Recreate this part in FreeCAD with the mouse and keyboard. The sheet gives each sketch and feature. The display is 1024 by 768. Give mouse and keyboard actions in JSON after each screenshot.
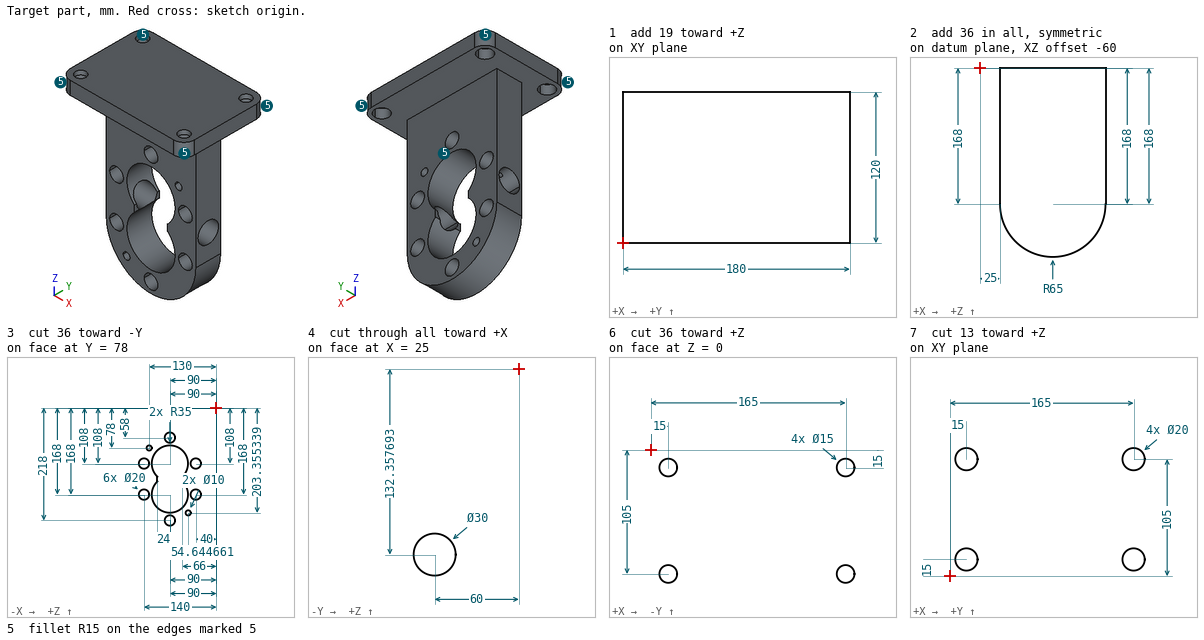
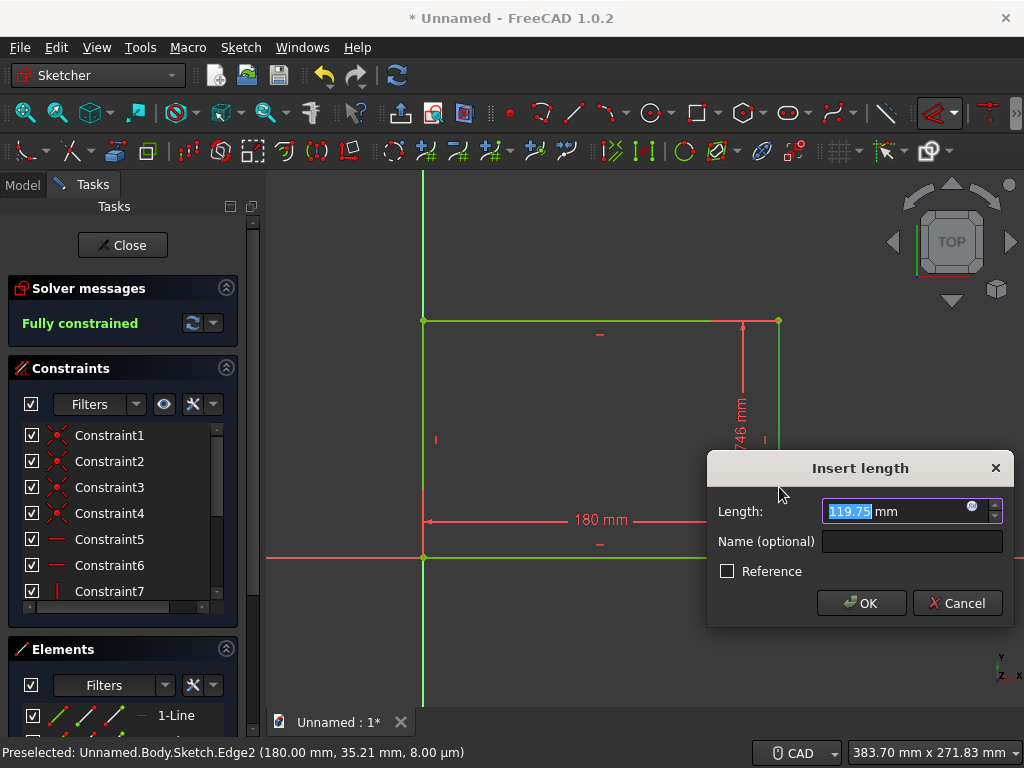
{"action": "type", "text": "120"}
{"action": "key", "text": "Return"}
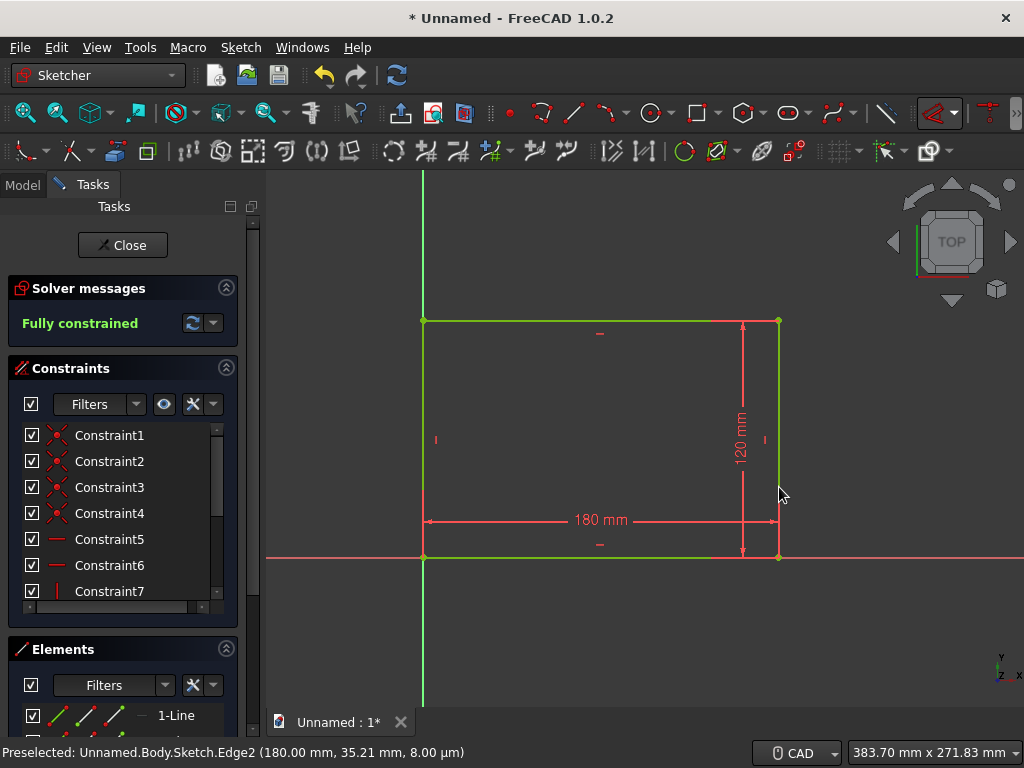
{"action": "left_click", "coordinate": [123, 245]}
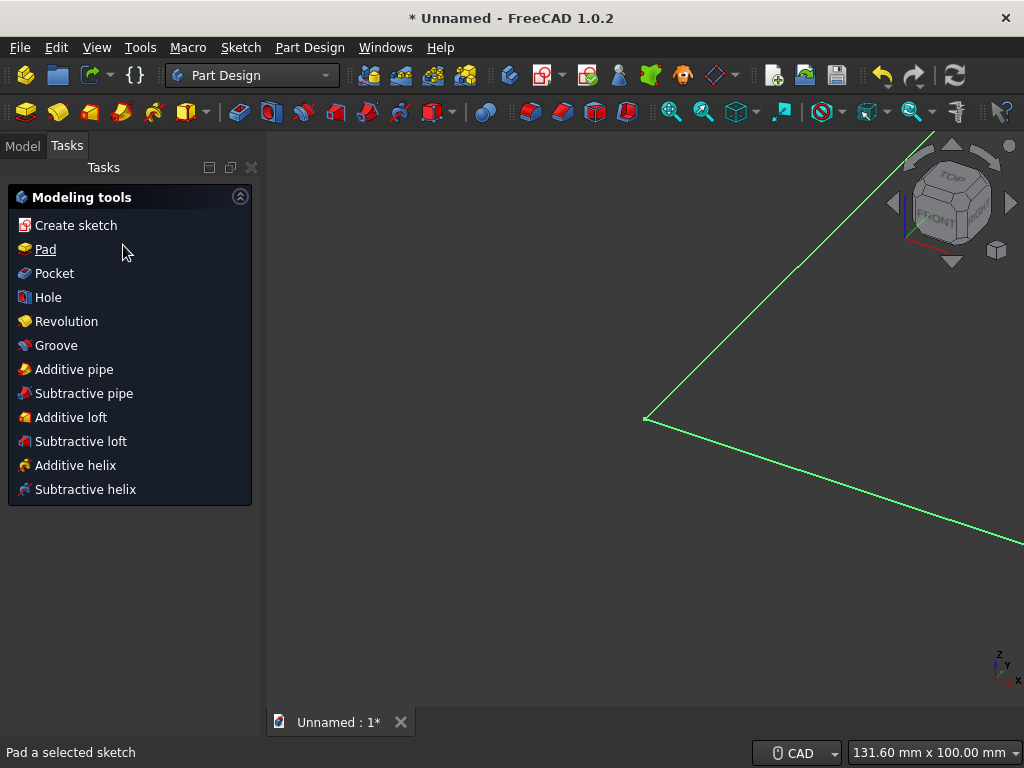
{"action": "left_click", "coordinate": [26, 112]}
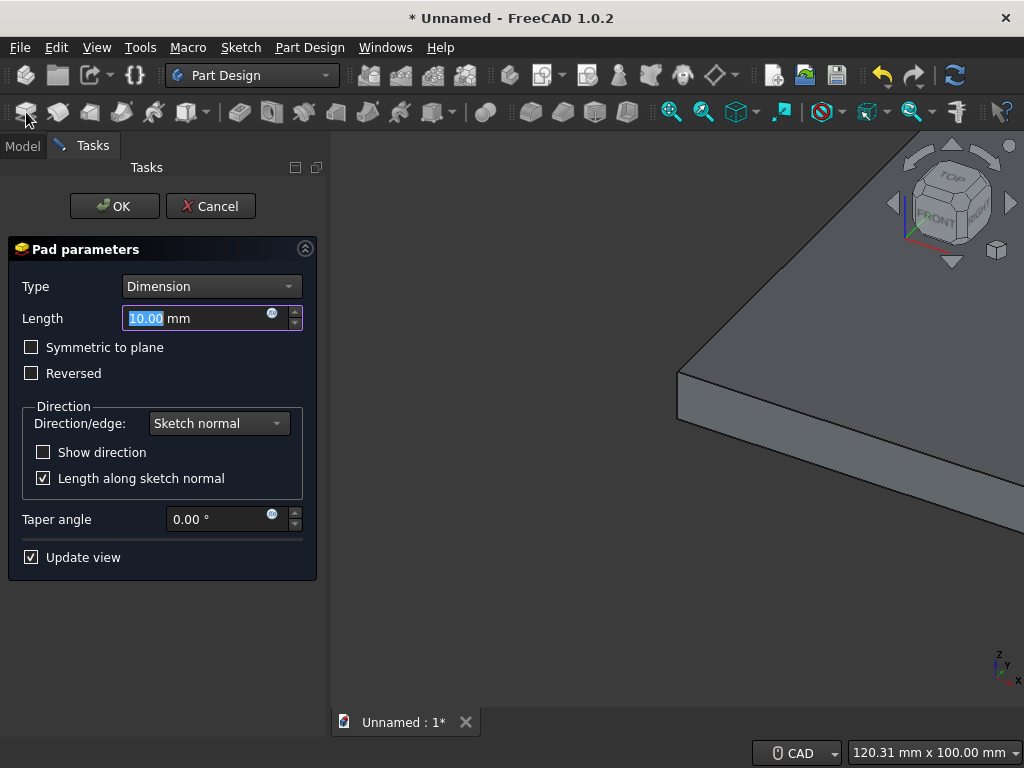
{"action": "type", "text": "19"}
{"action": "key", "text": "Tab"}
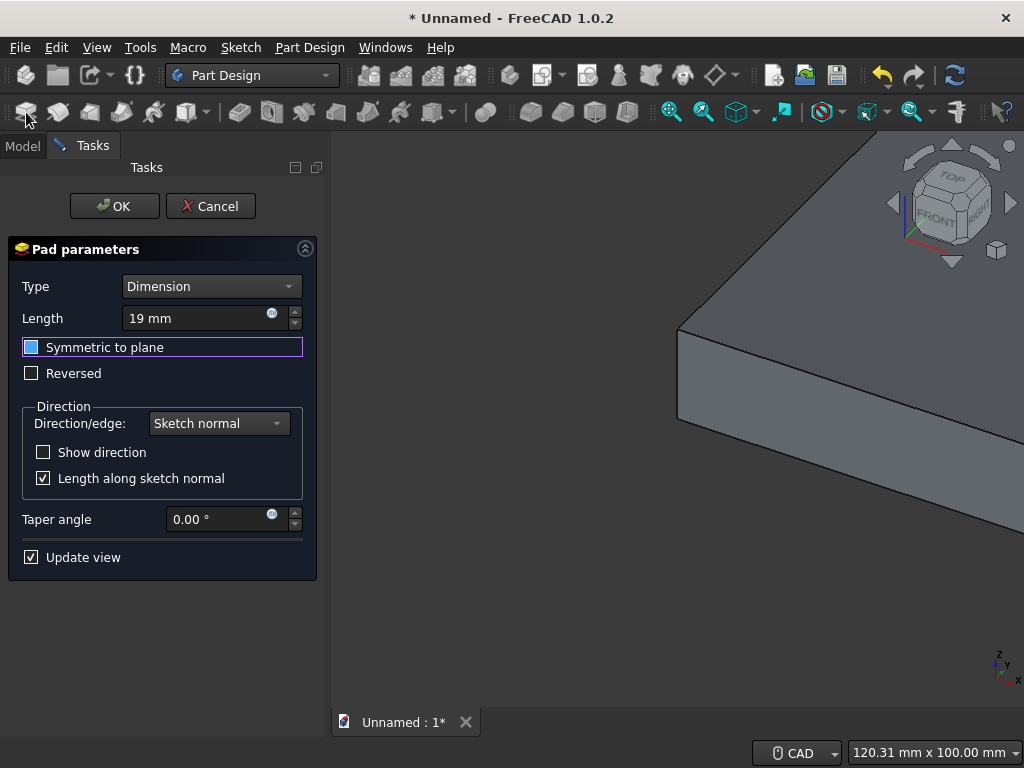
{"action": "left_click", "coordinate": [115, 206]}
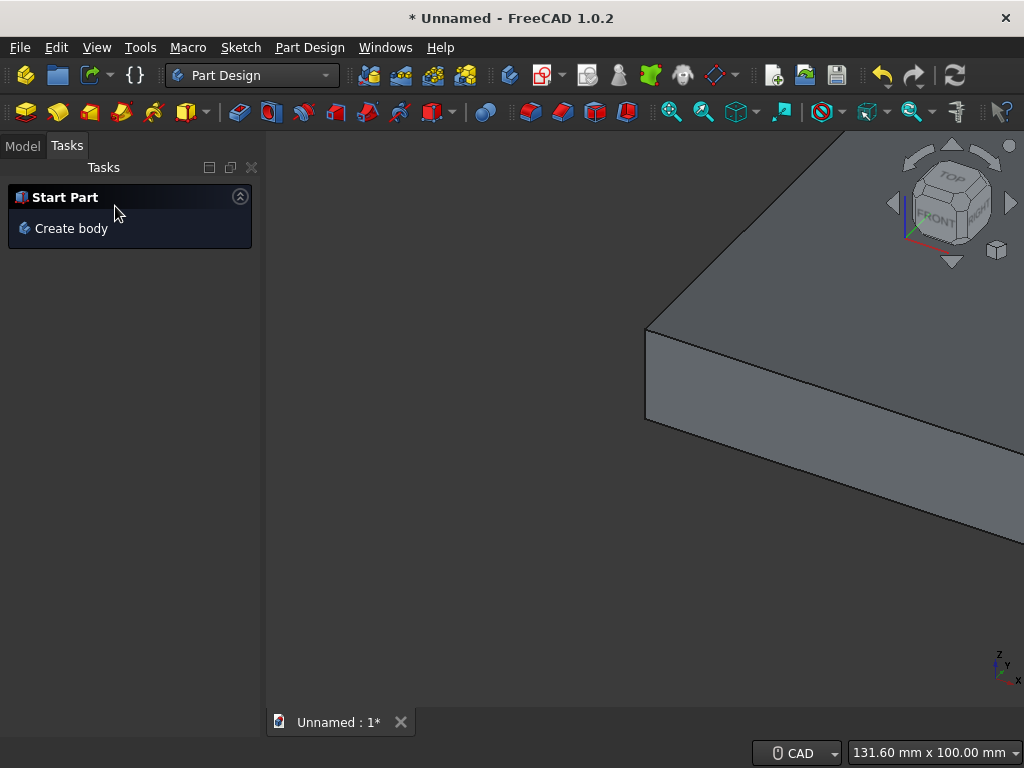
{"action": "left_click", "coordinate": [672, 112]}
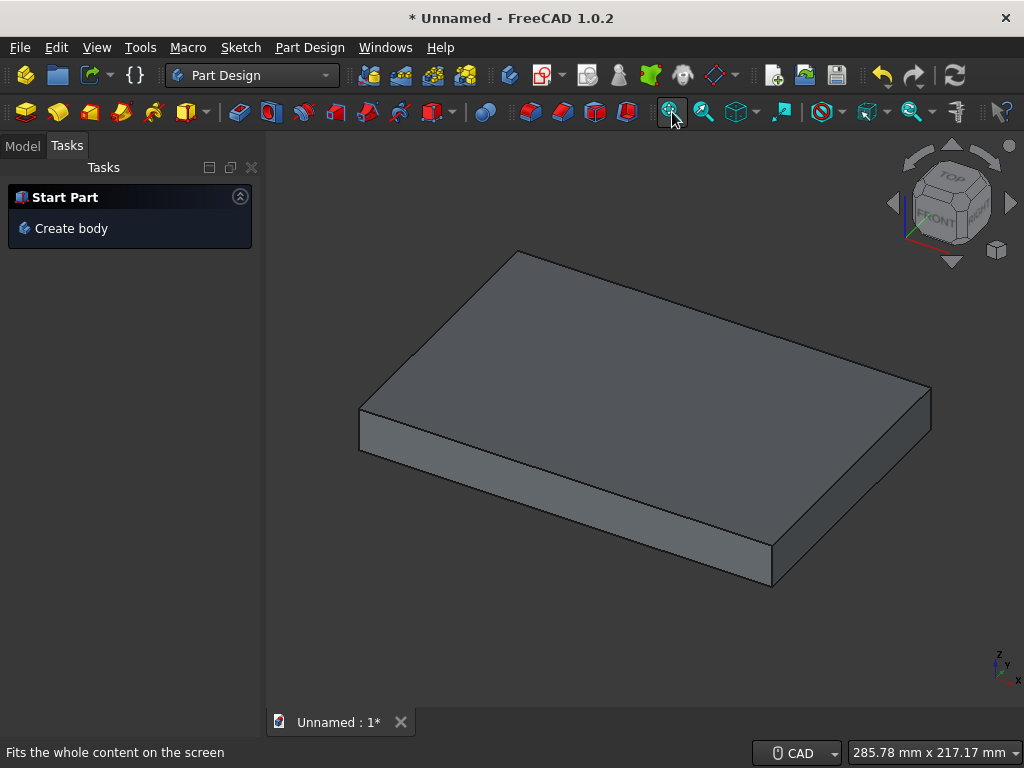
{"action": "left_click", "coordinate": [23, 145]}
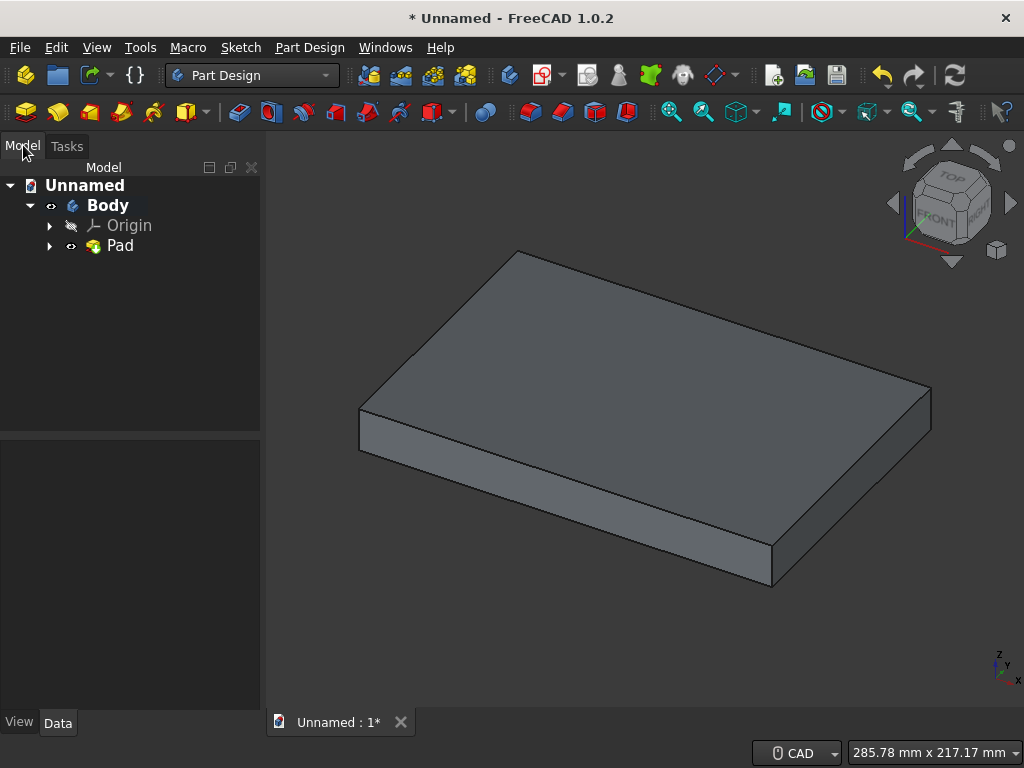
{"action": "left_click", "coordinate": [50, 226]}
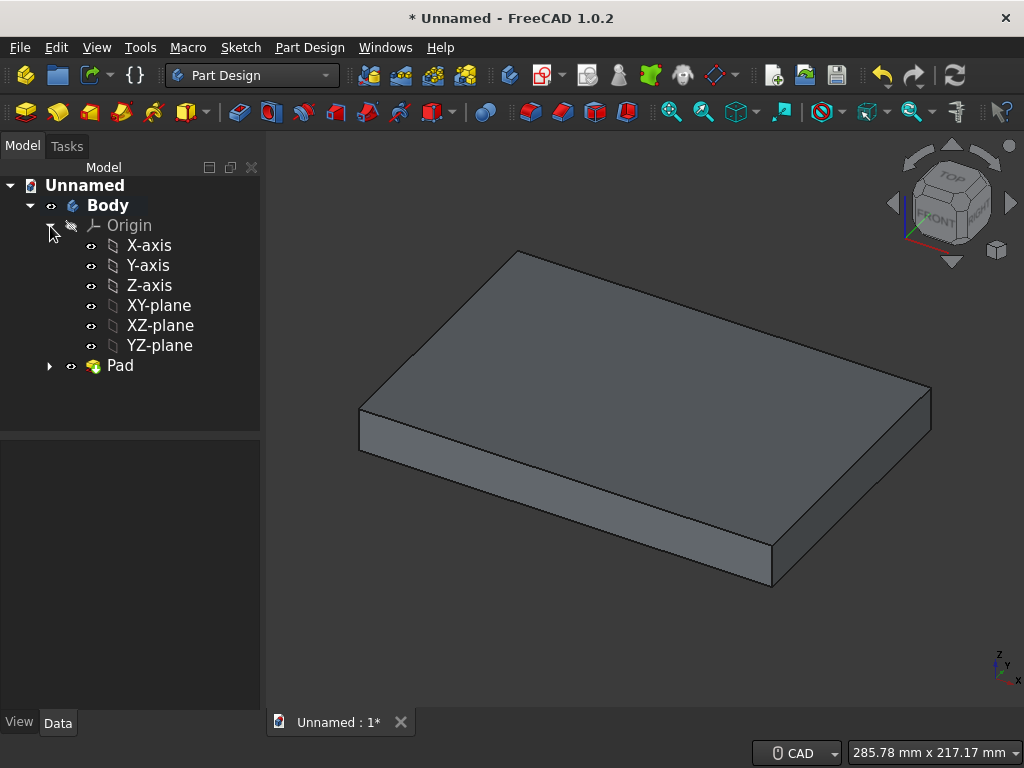
{"action": "left_click", "coordinate": [136, 326]}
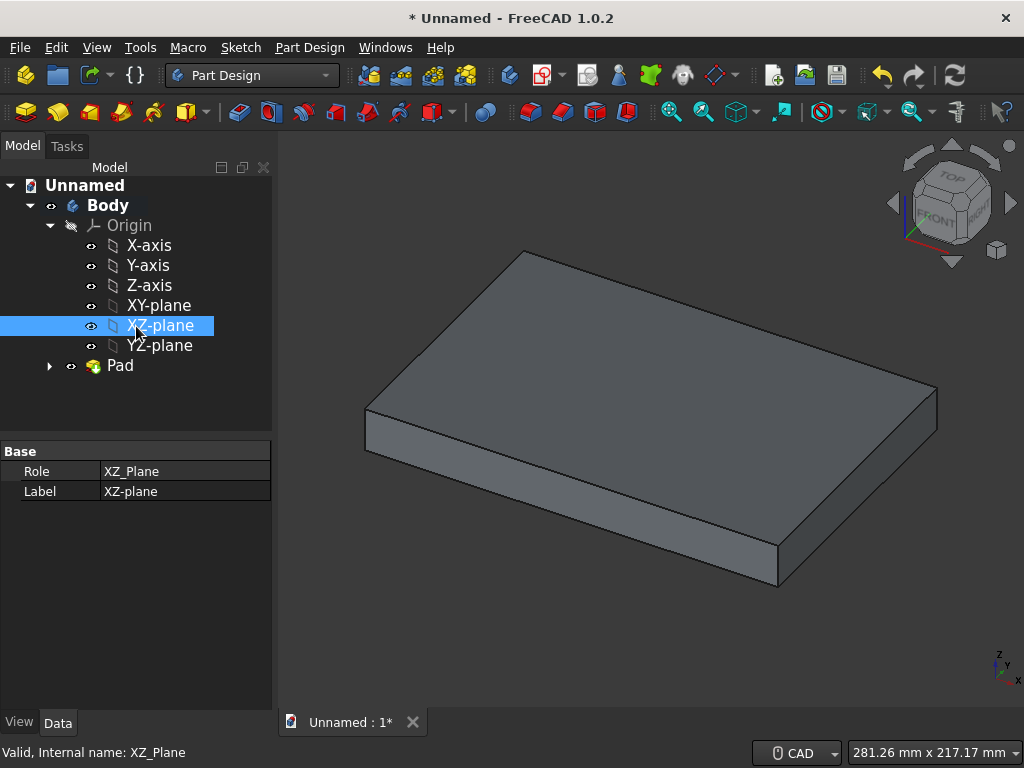
{"action": "left_click", "coordinate": [716, 76]}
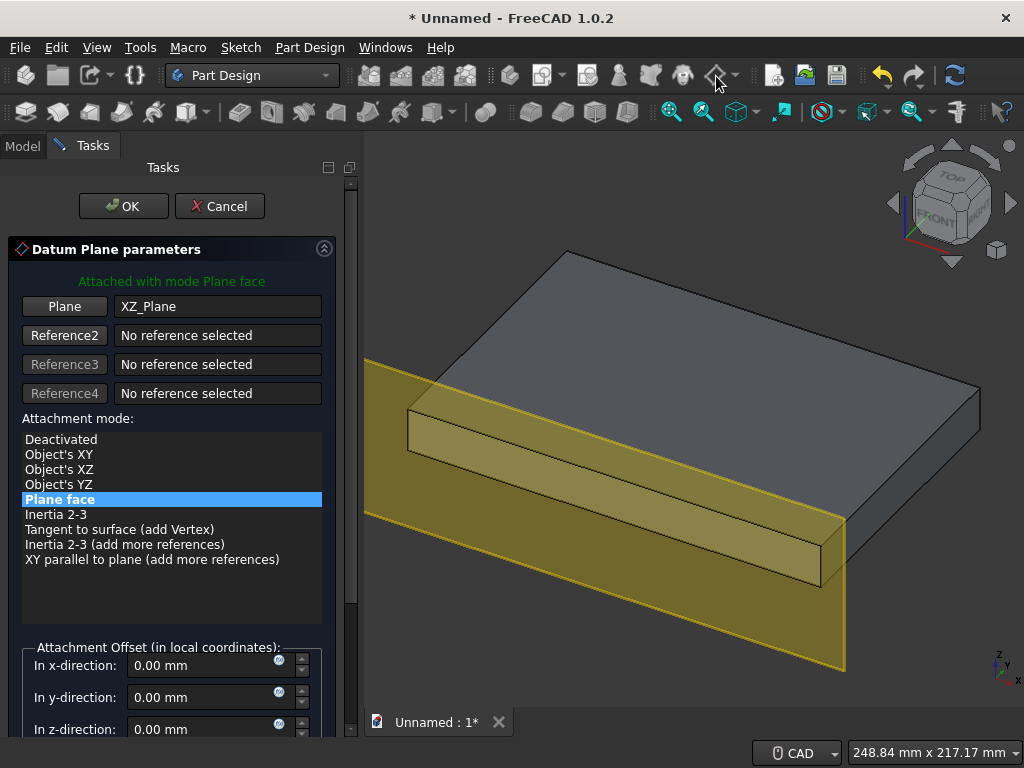
{"action": "scroll", "coordinate": [351, 456], "scroll_direction": "down", "scroll_amount": 2}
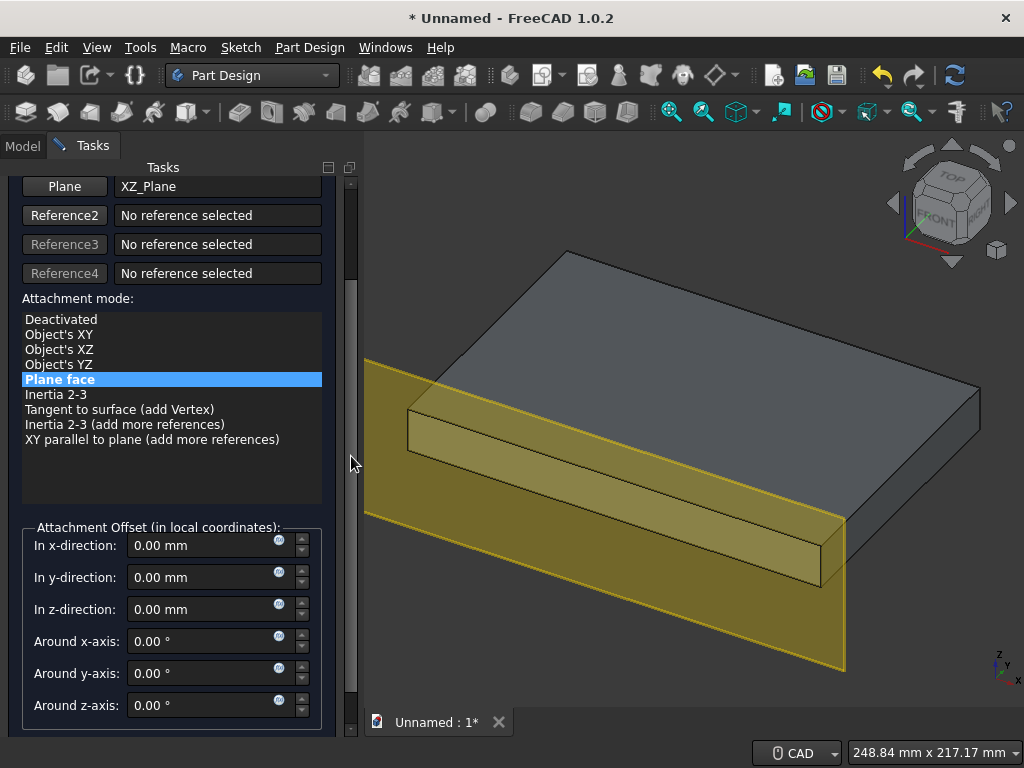
{"action": "triple_click", "coordinate": [210, 609]}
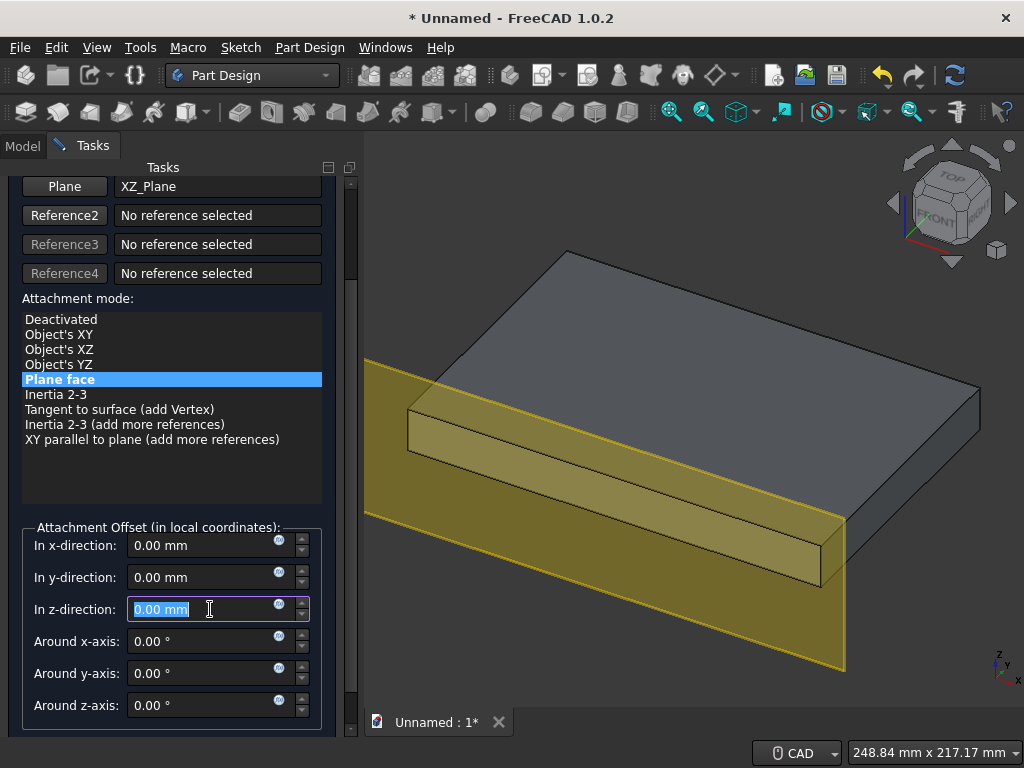
{"action": "type", "text": "-60"}
{"action": "key", "text": "Tab"}